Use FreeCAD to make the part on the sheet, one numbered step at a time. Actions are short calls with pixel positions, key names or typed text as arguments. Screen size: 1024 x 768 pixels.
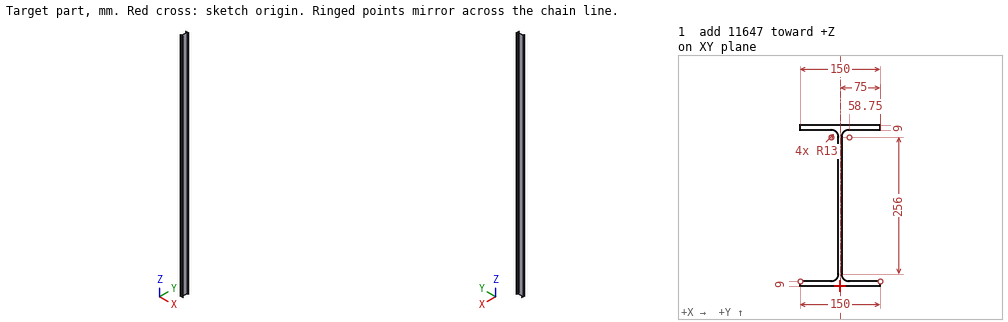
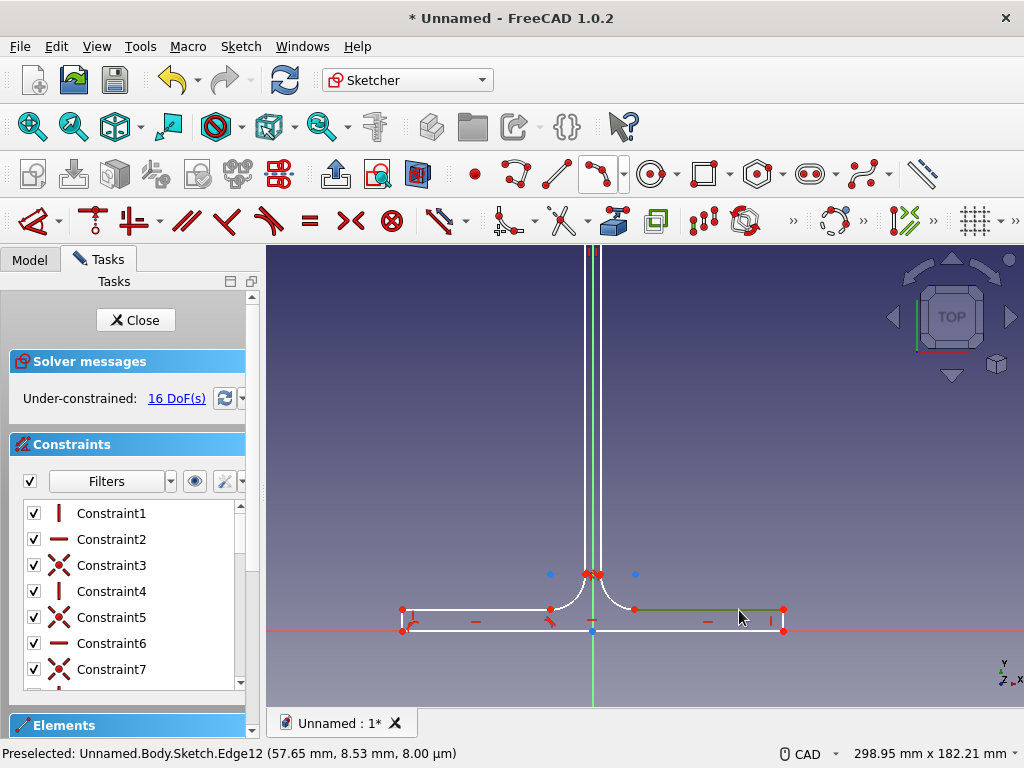
click(605, 590)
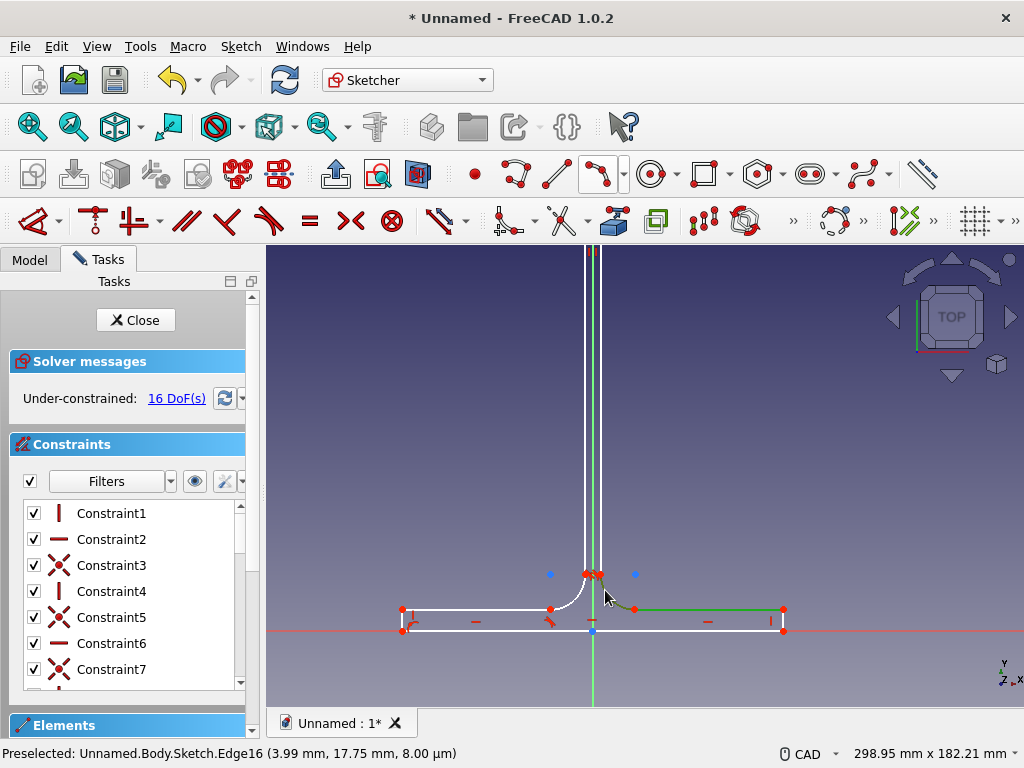
key(t)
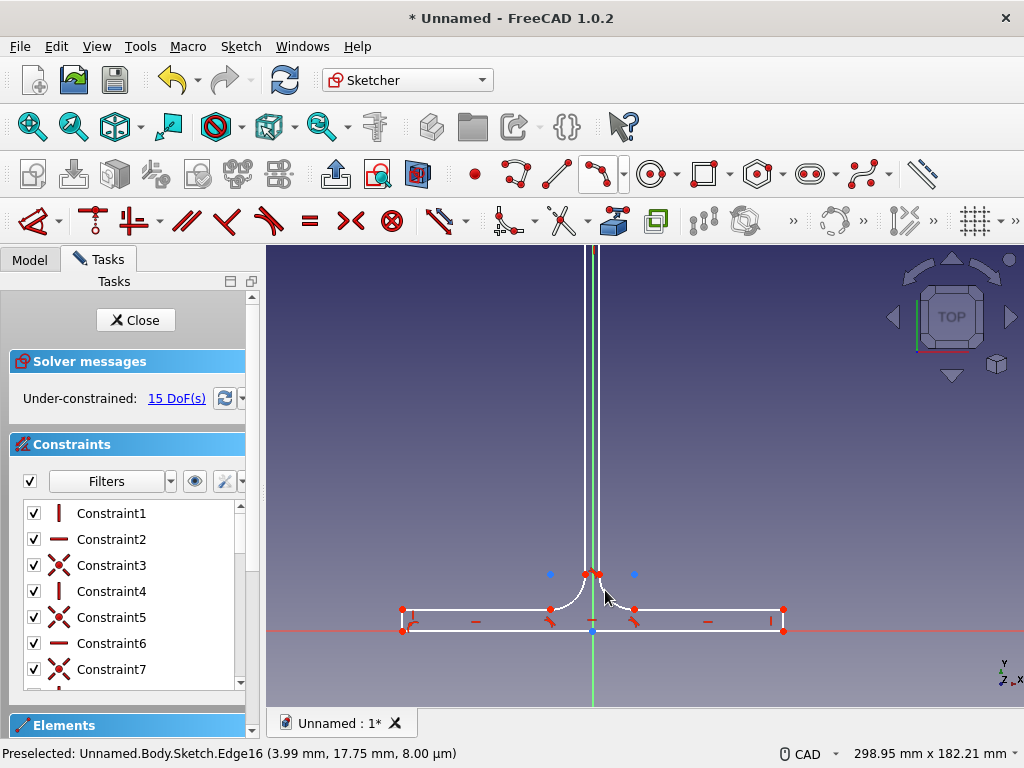
scroll(567, 607, down, 5)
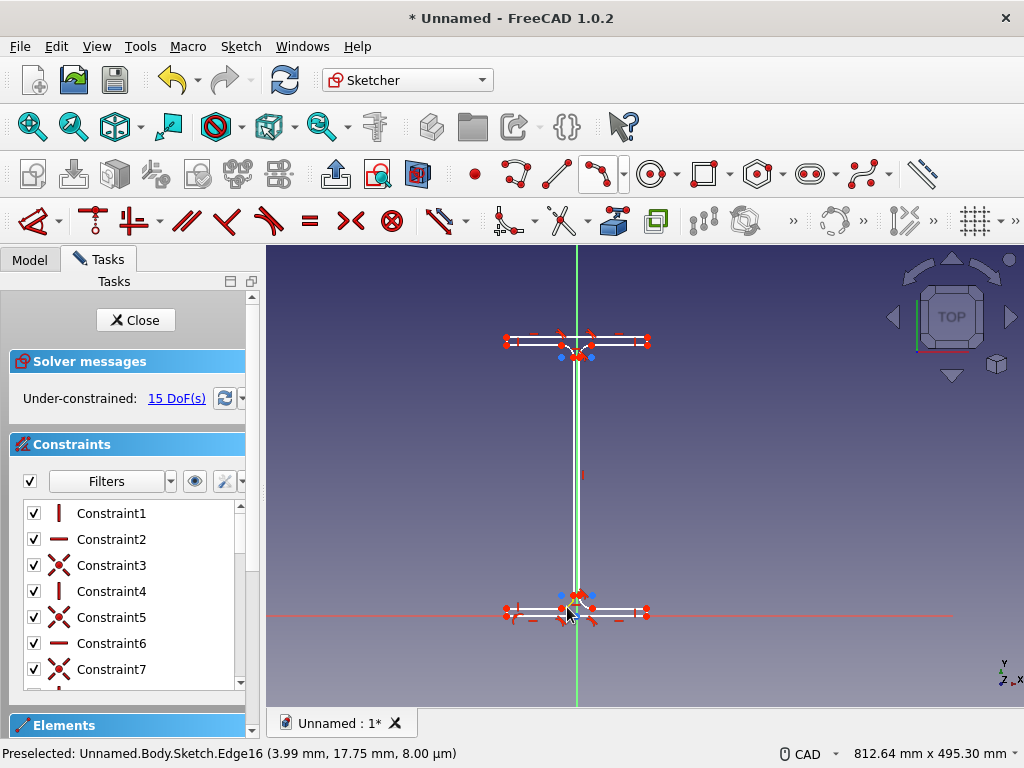
scroll(586, 346, up, 5)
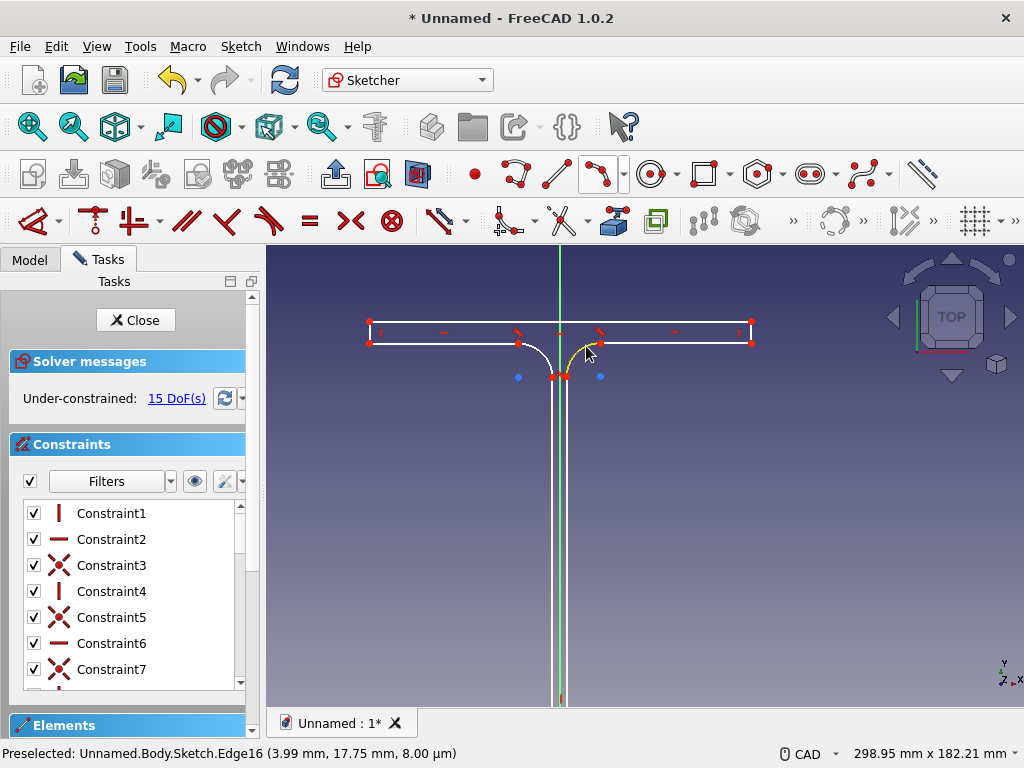
click(585, 347)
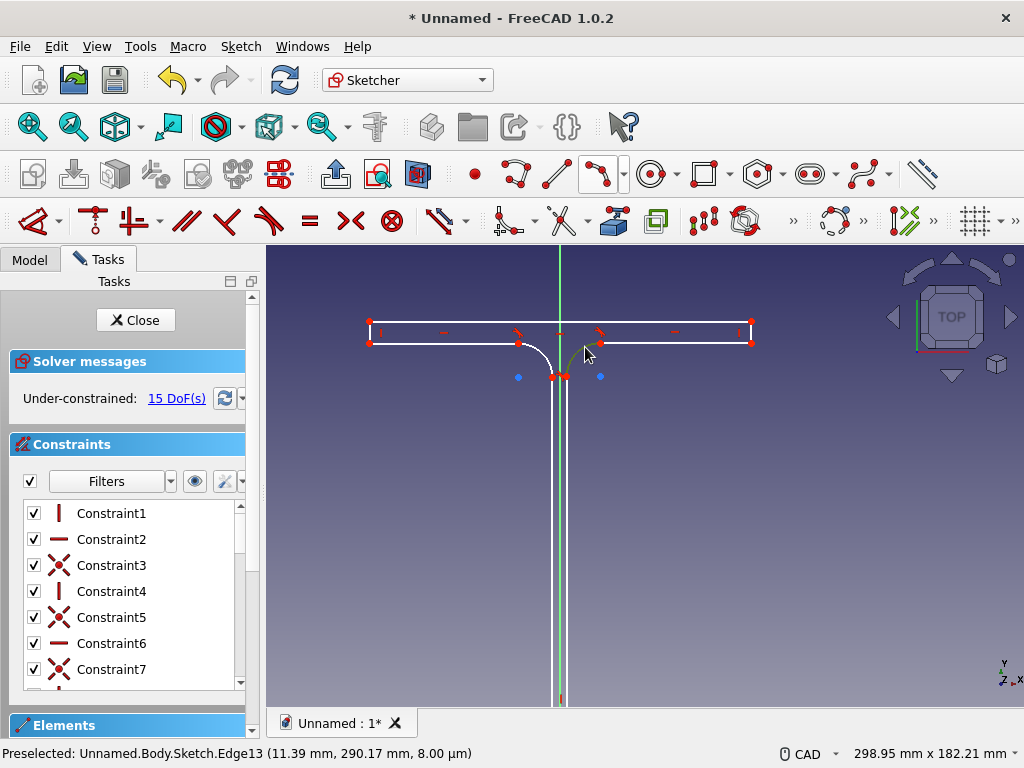
click(549, 362)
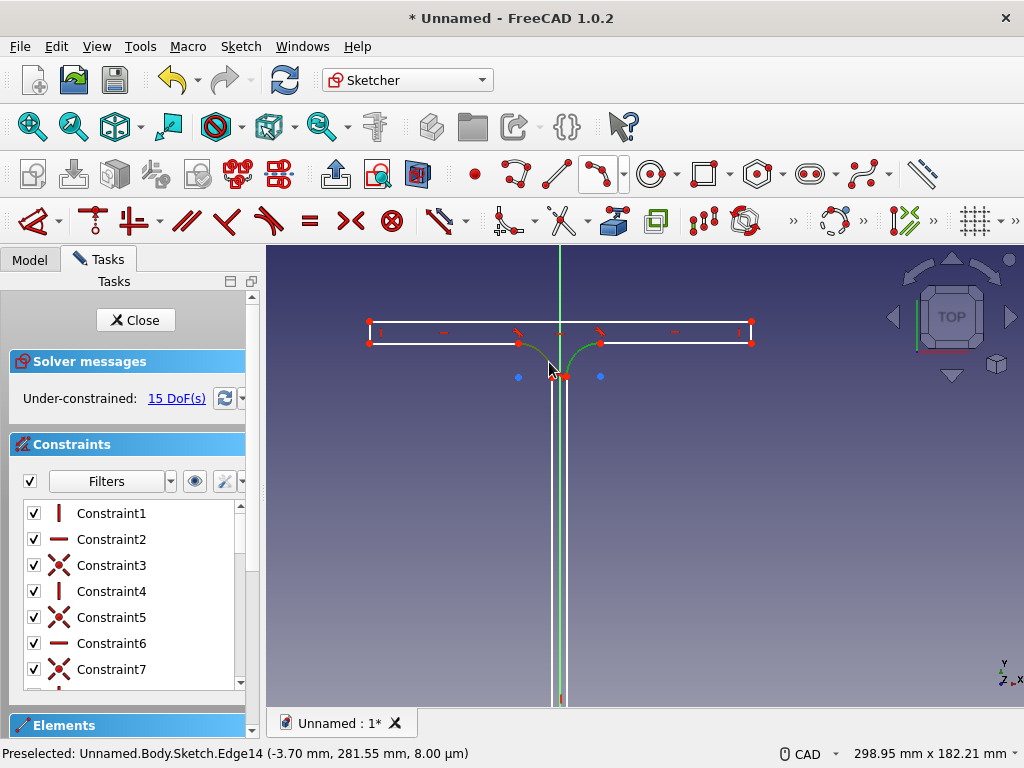
scroll(586, 345, down, 5)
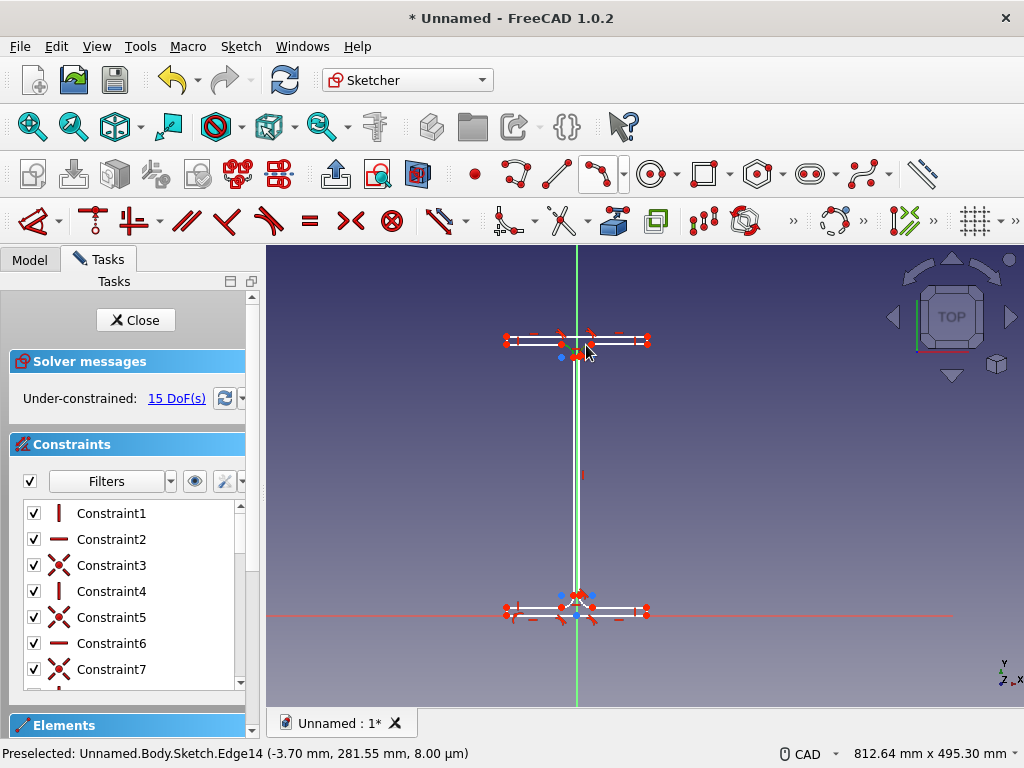
scroll(567, 606, up, 5)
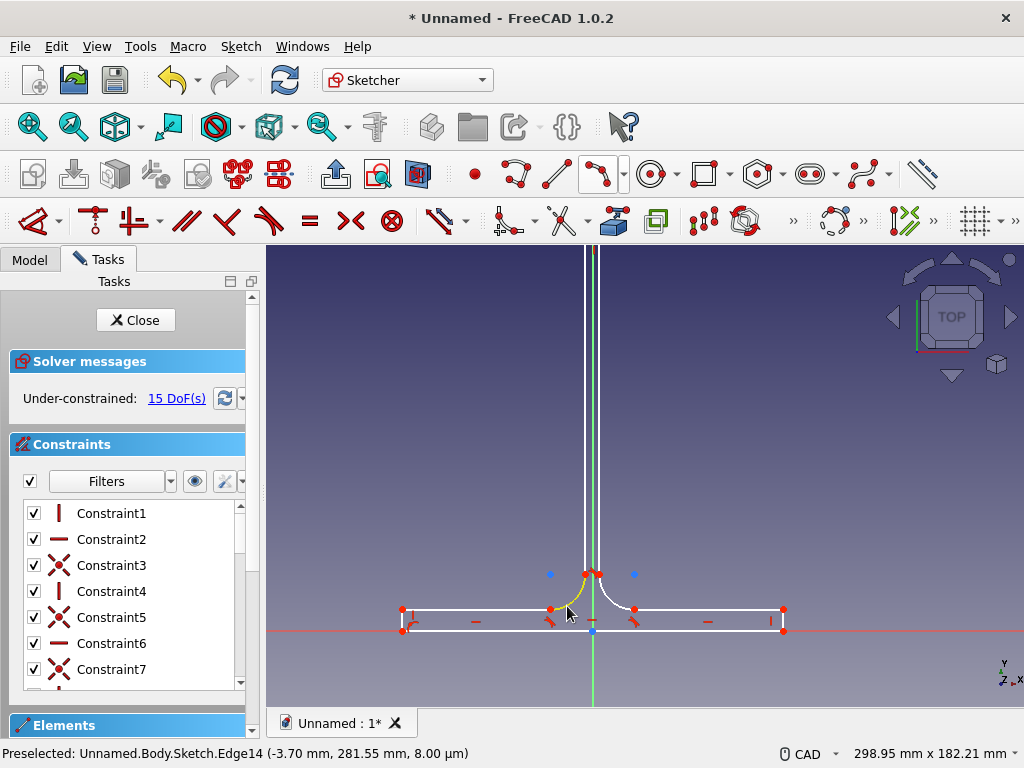
click(566, 606)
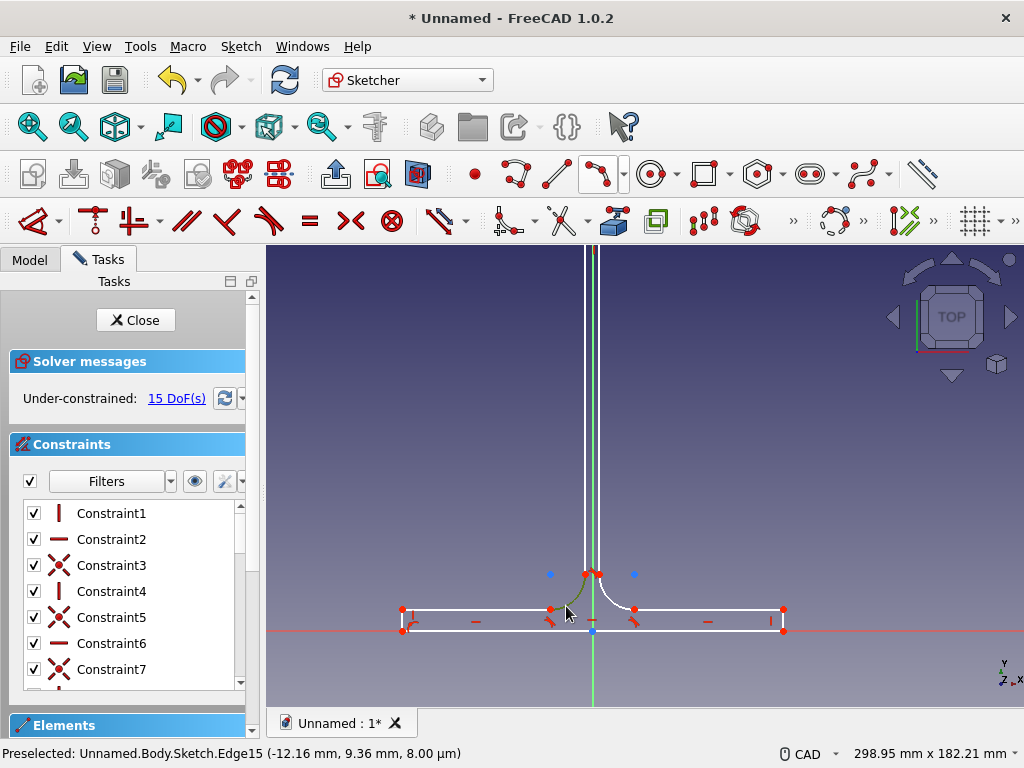
scroll(603, 591, up, 2)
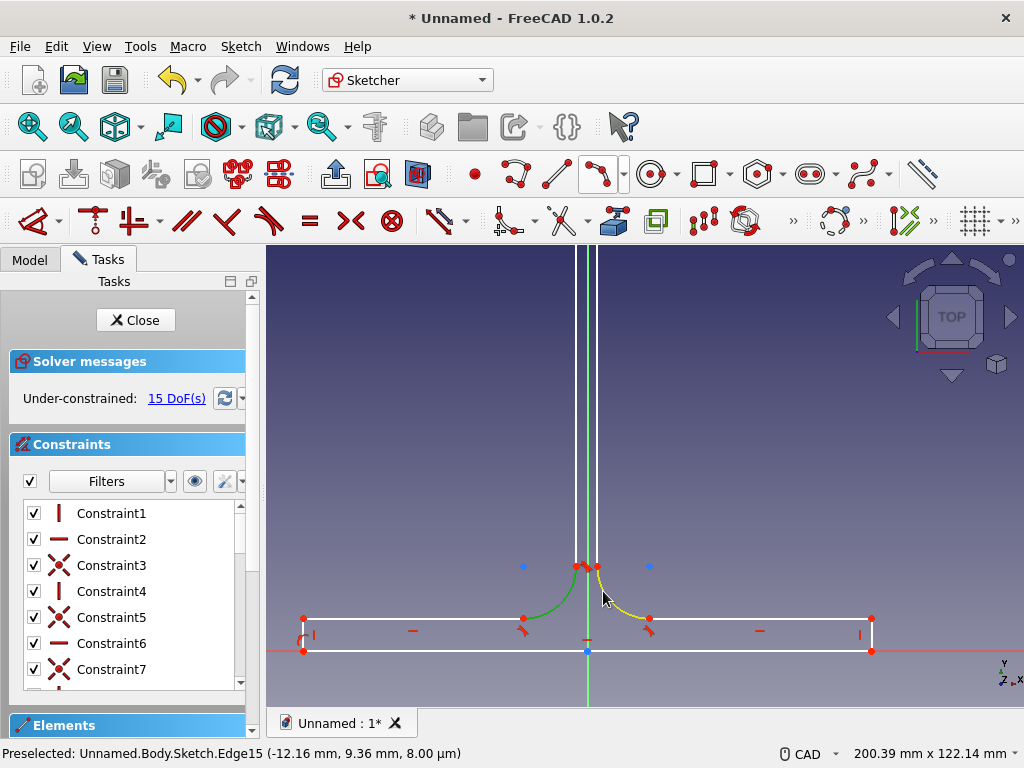
click(603, 590)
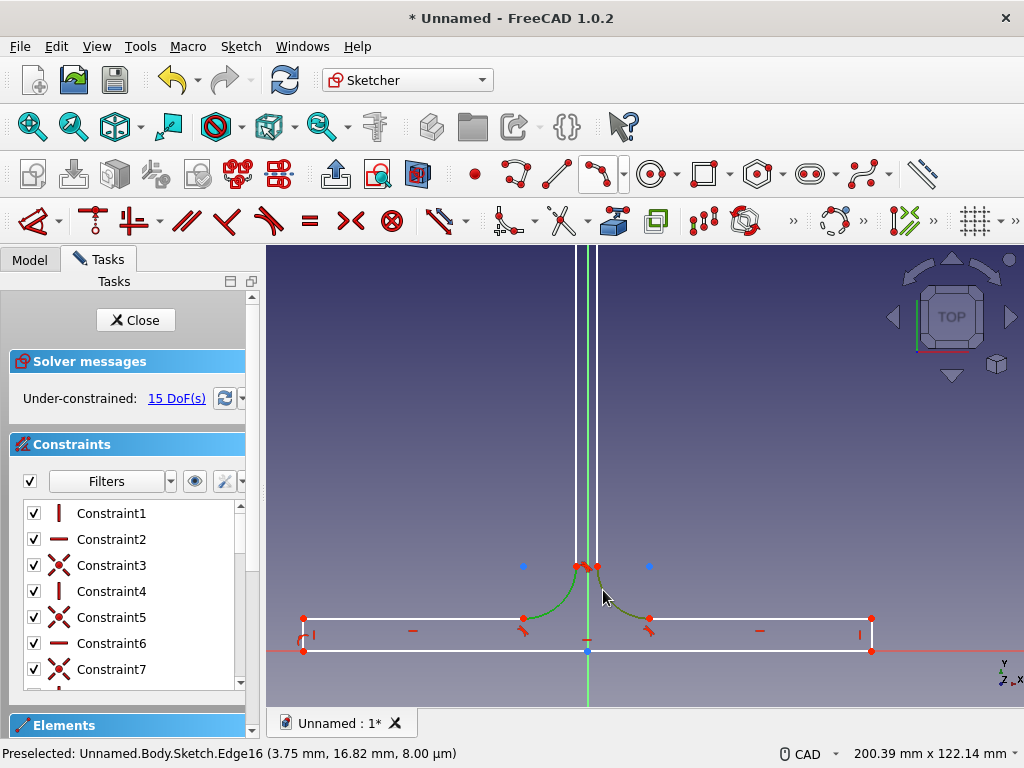
key(e)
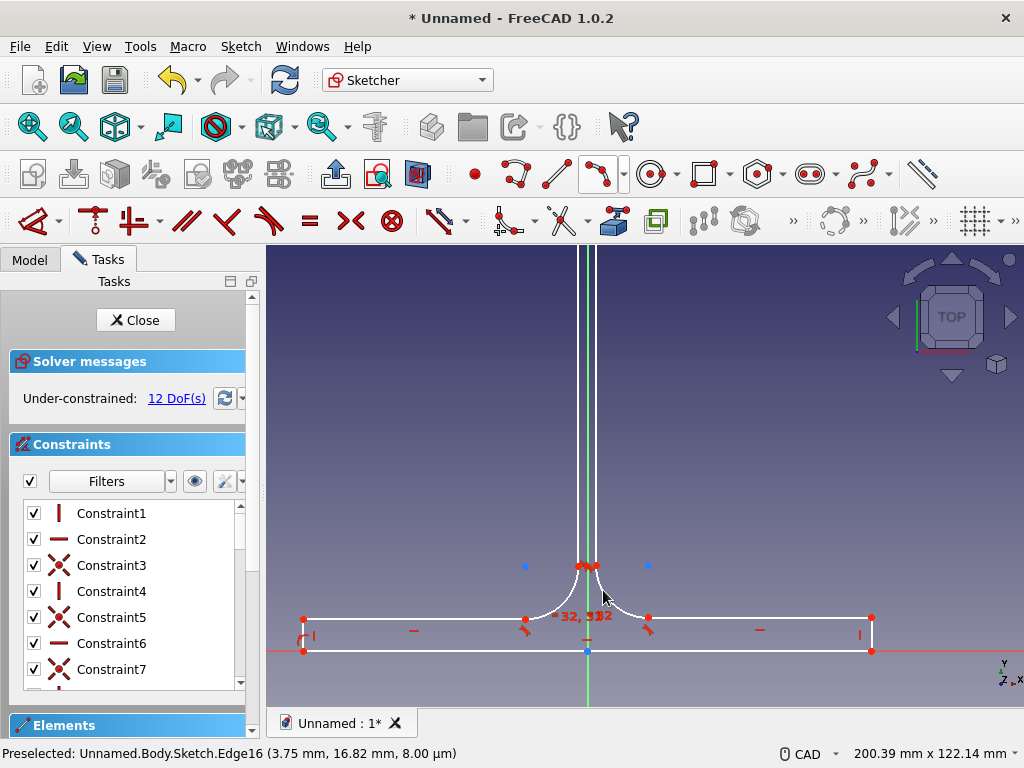
scroll(573, 604, down, 7)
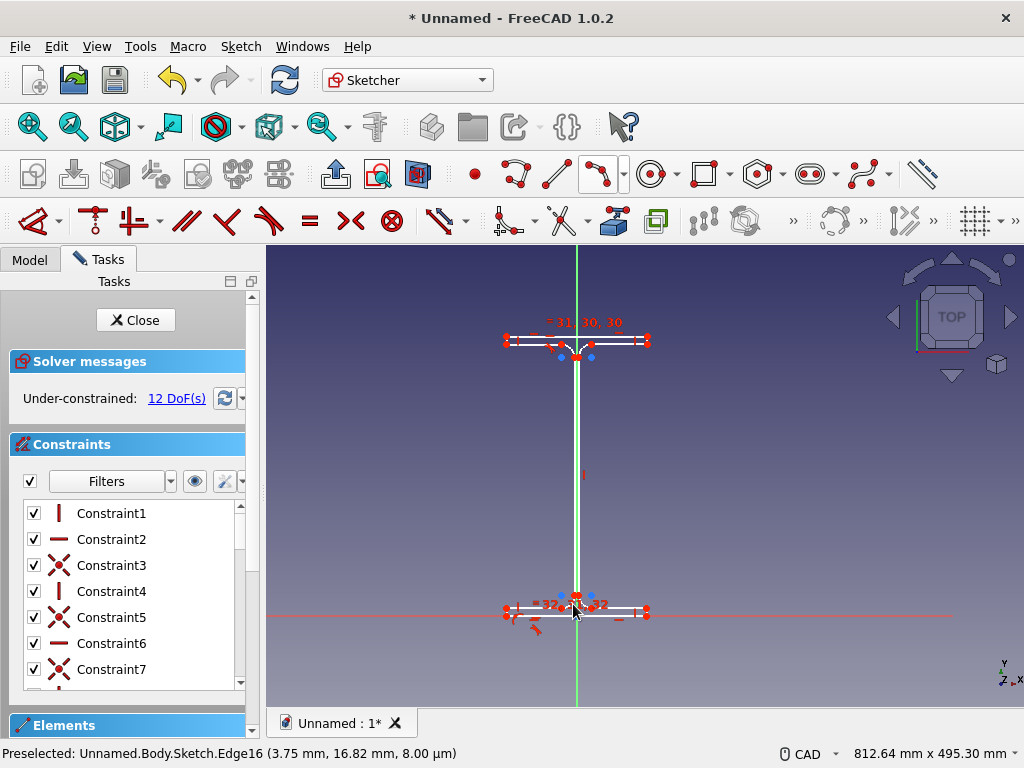
click(592, 357)